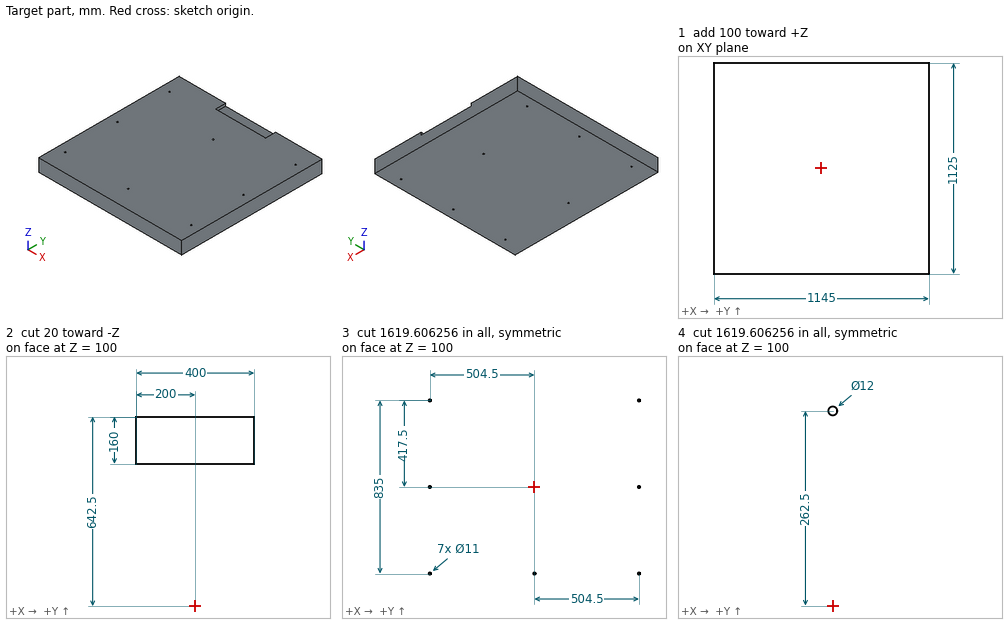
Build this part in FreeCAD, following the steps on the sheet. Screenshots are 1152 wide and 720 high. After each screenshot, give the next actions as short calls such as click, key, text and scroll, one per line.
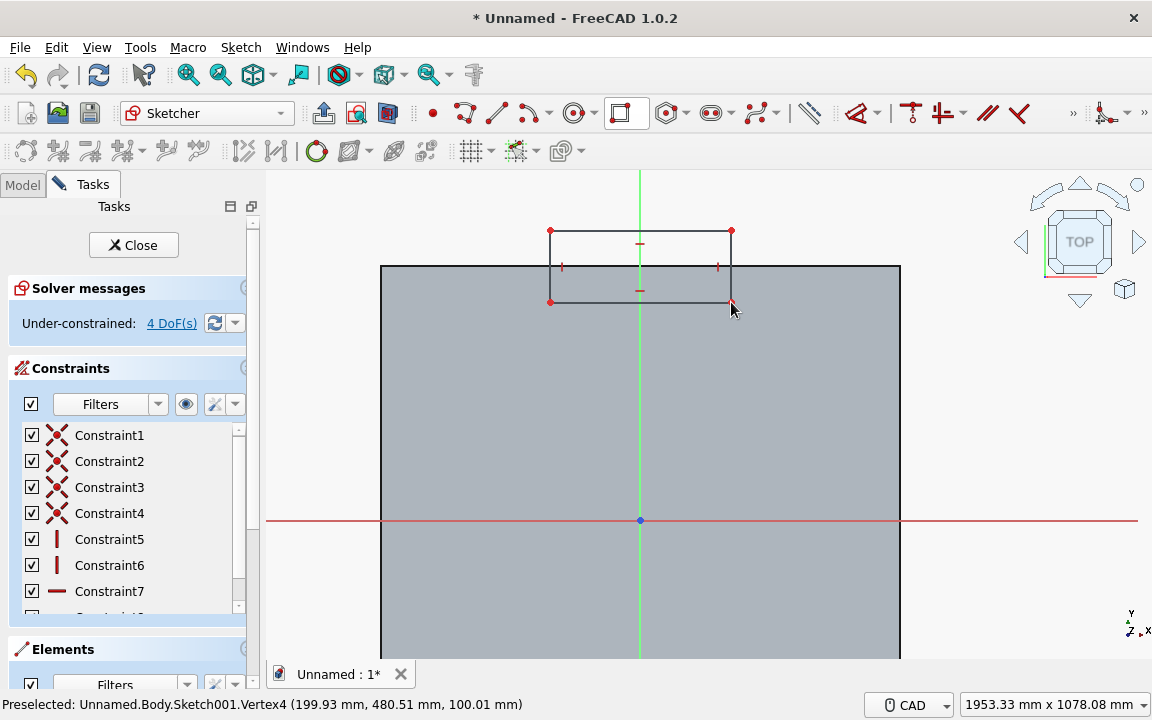
key(d)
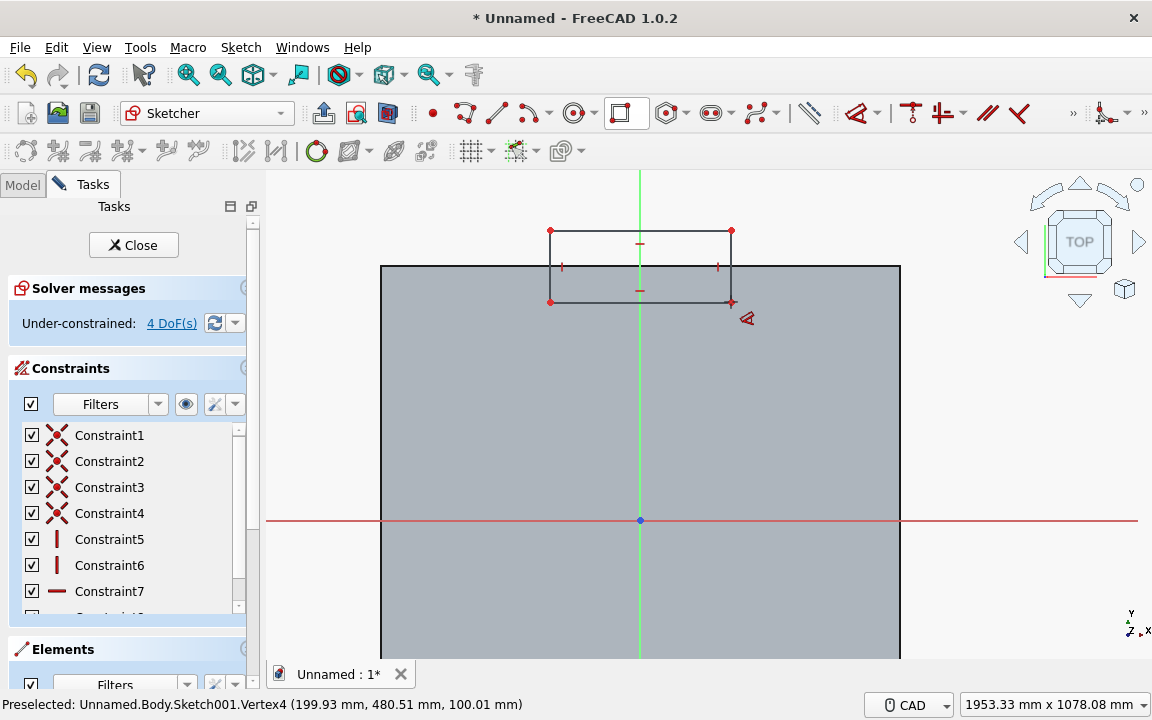
click(550, 253)
click(516, 267)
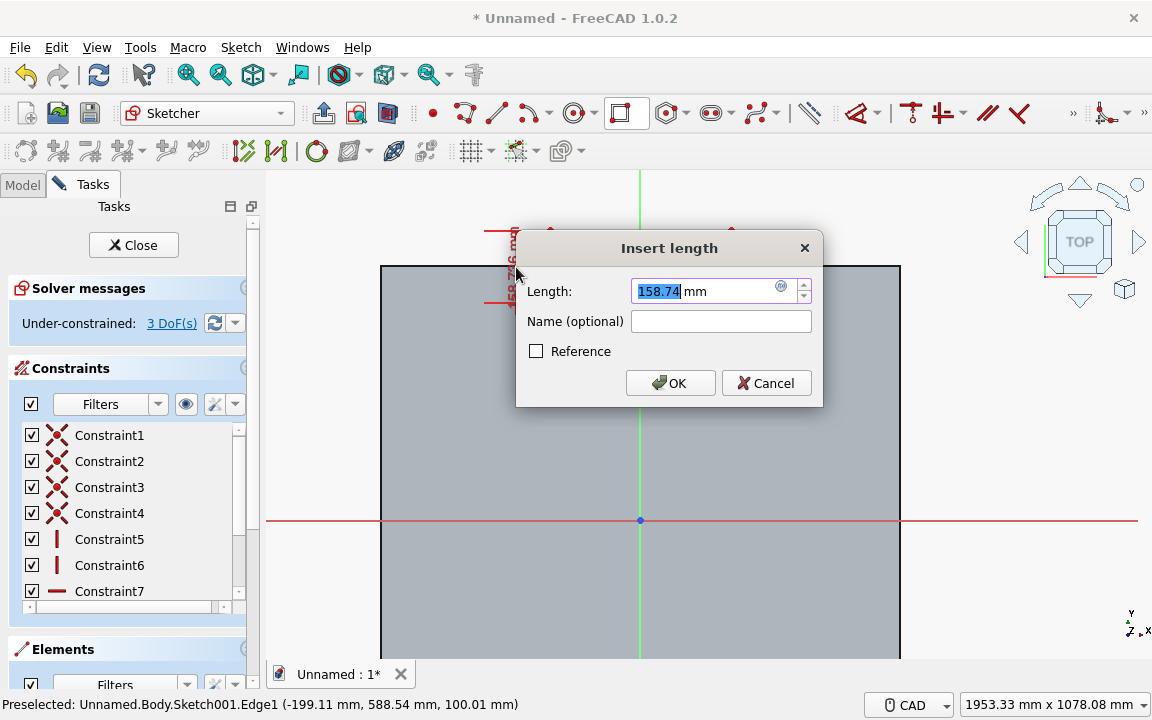
text(160)
key(Return)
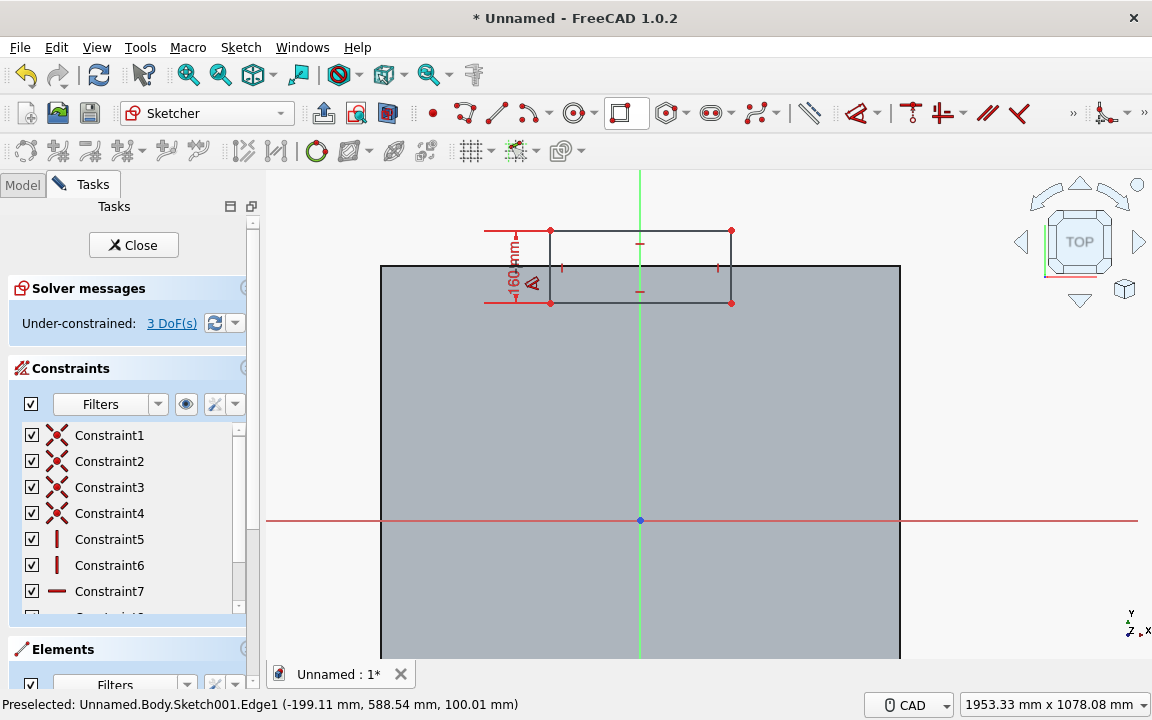
click(604, 303)
click(599, 269)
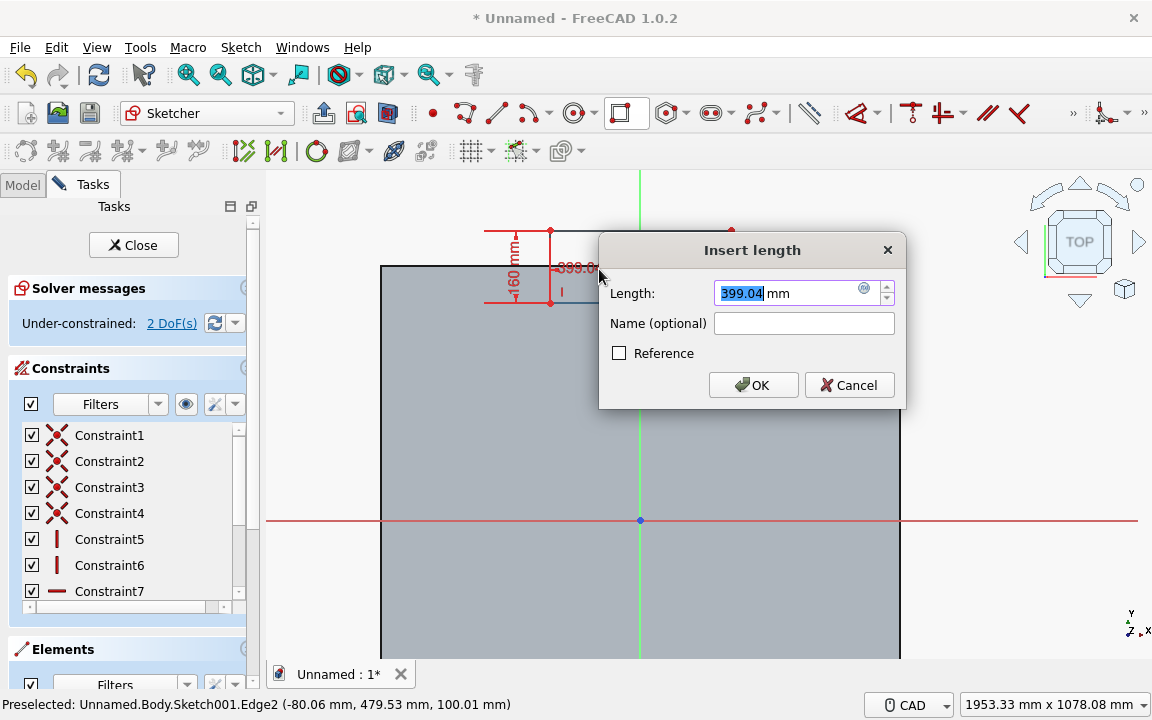
text(400)
key(Return)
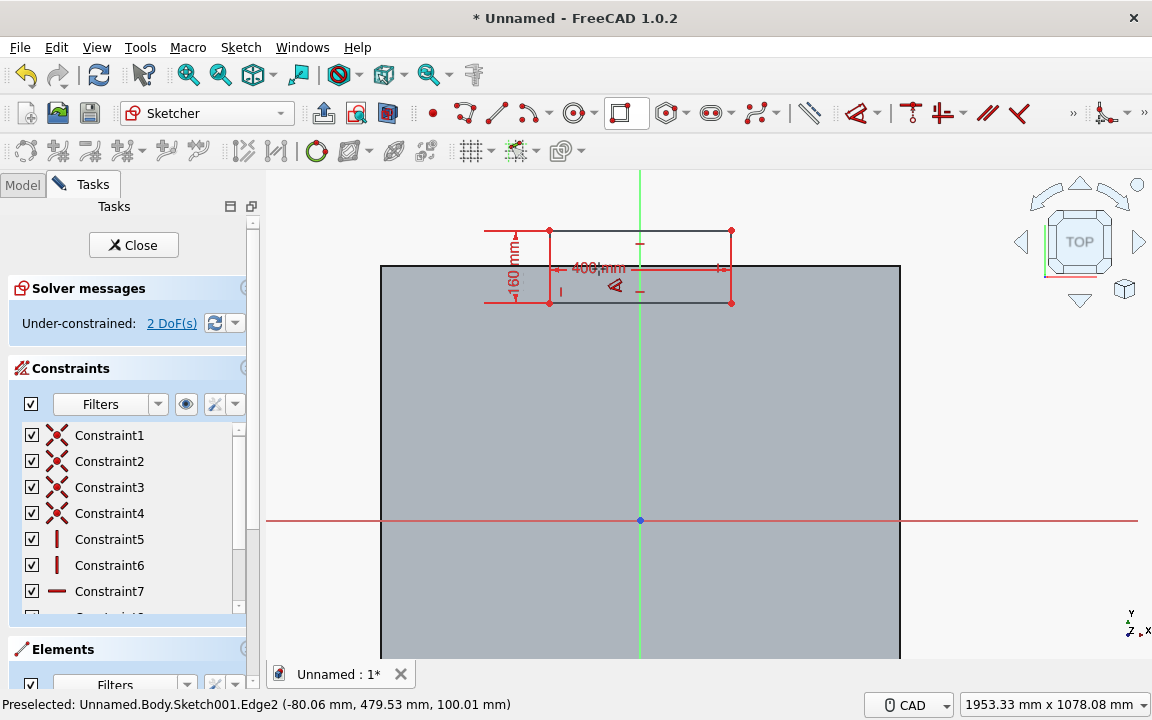
click(550, 231)
click(595, 555)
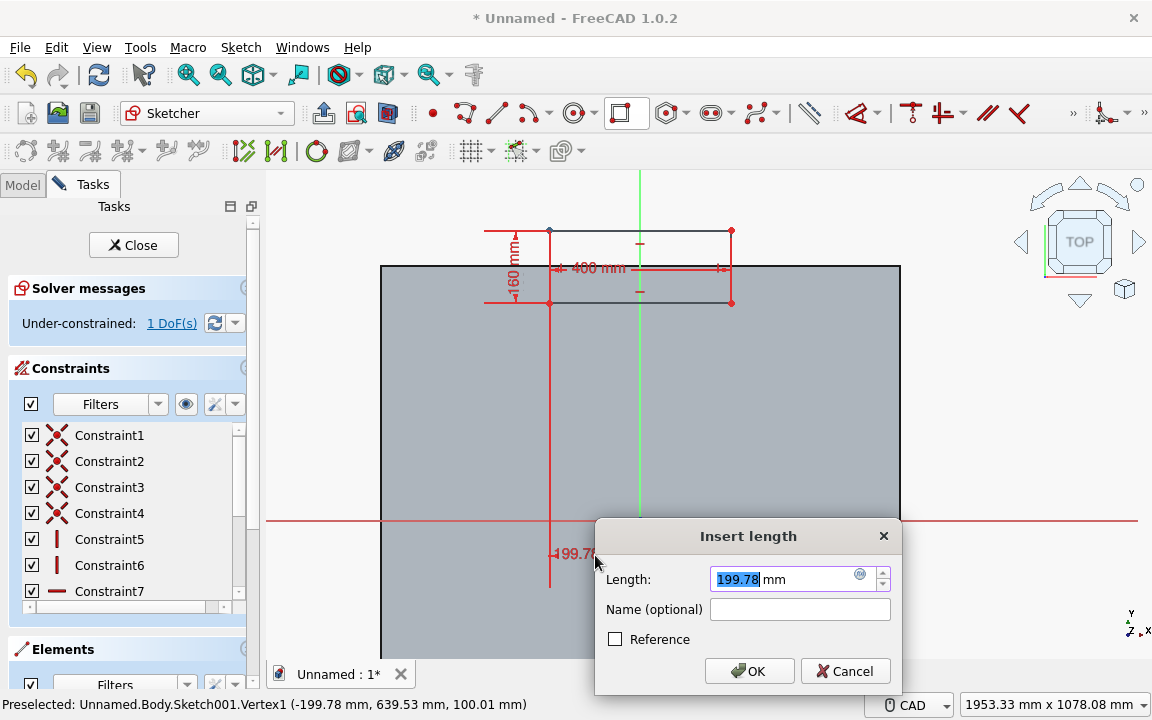
text(200)
key(Return)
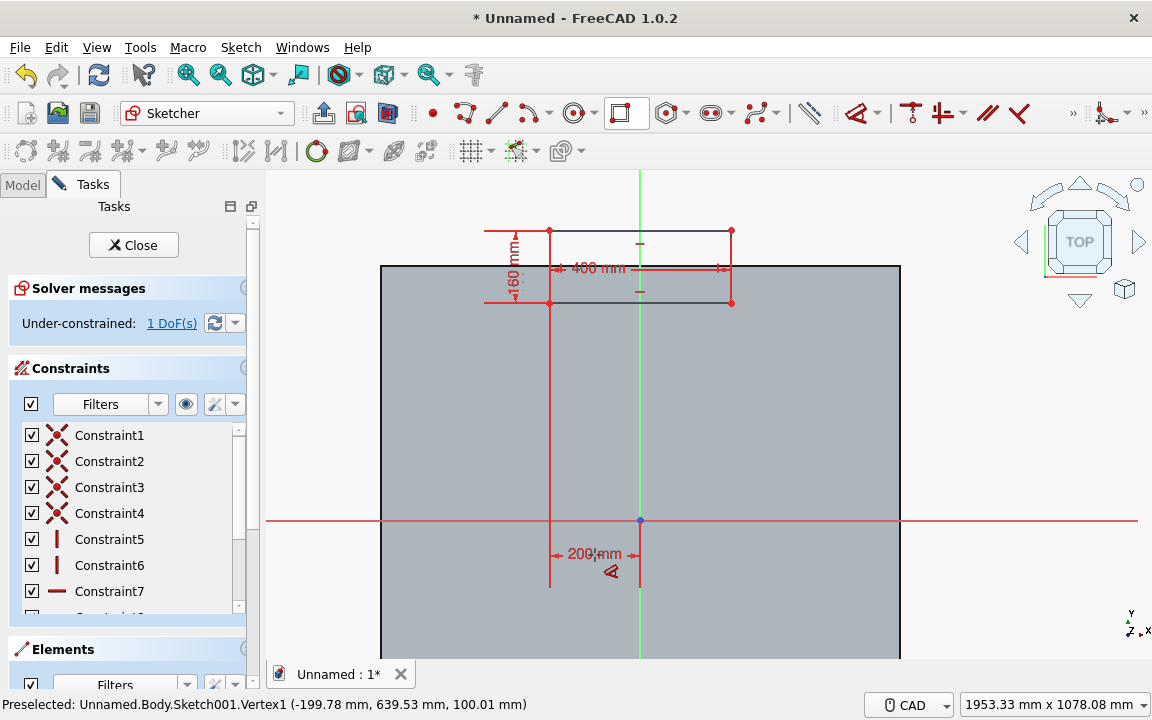
click(550, 231)
click(516, 376)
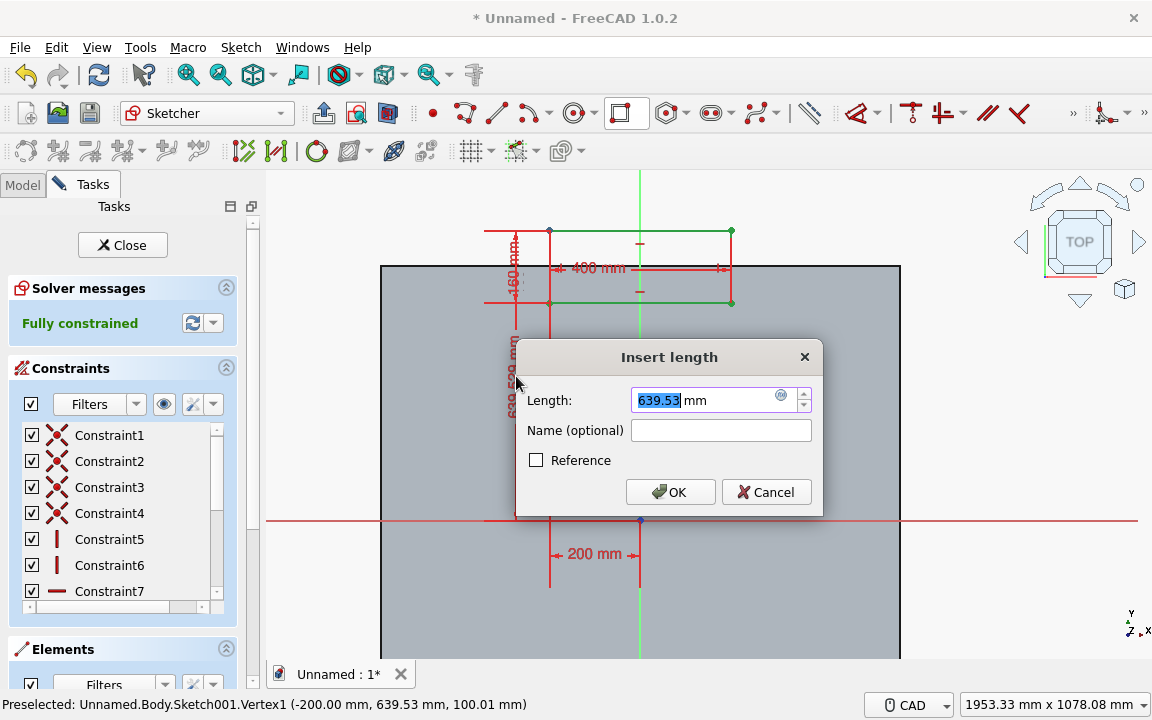
text(642.5)
key(Return)
key(Escape)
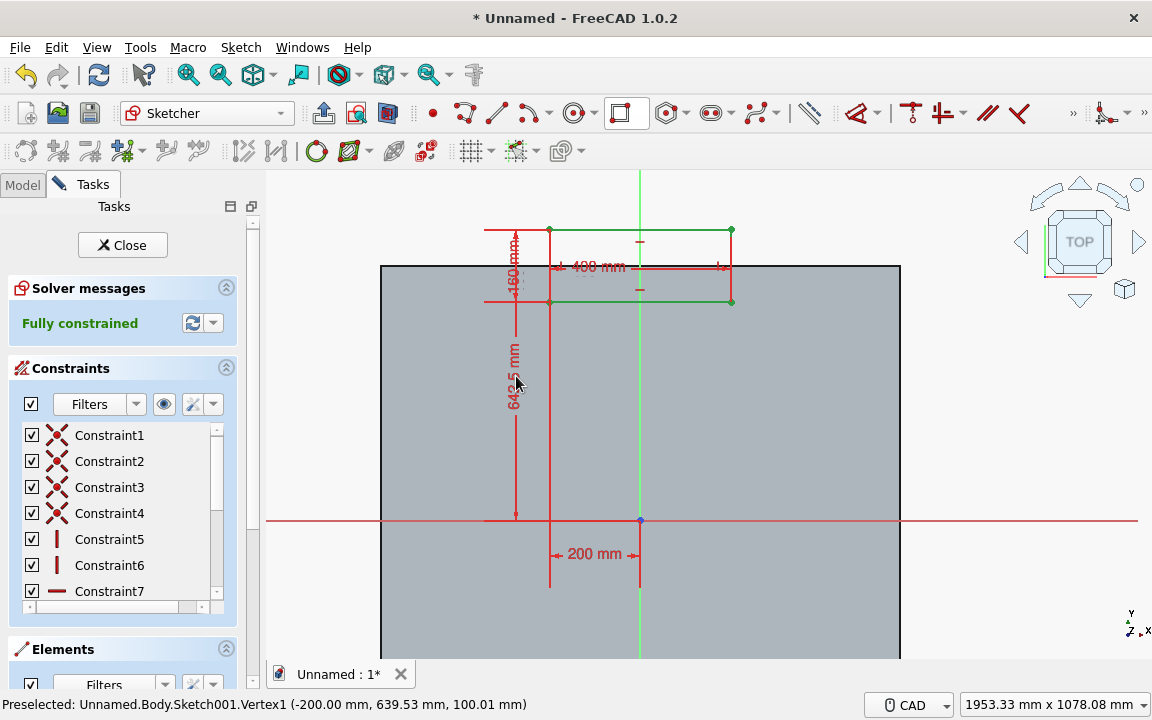
click(123, 245)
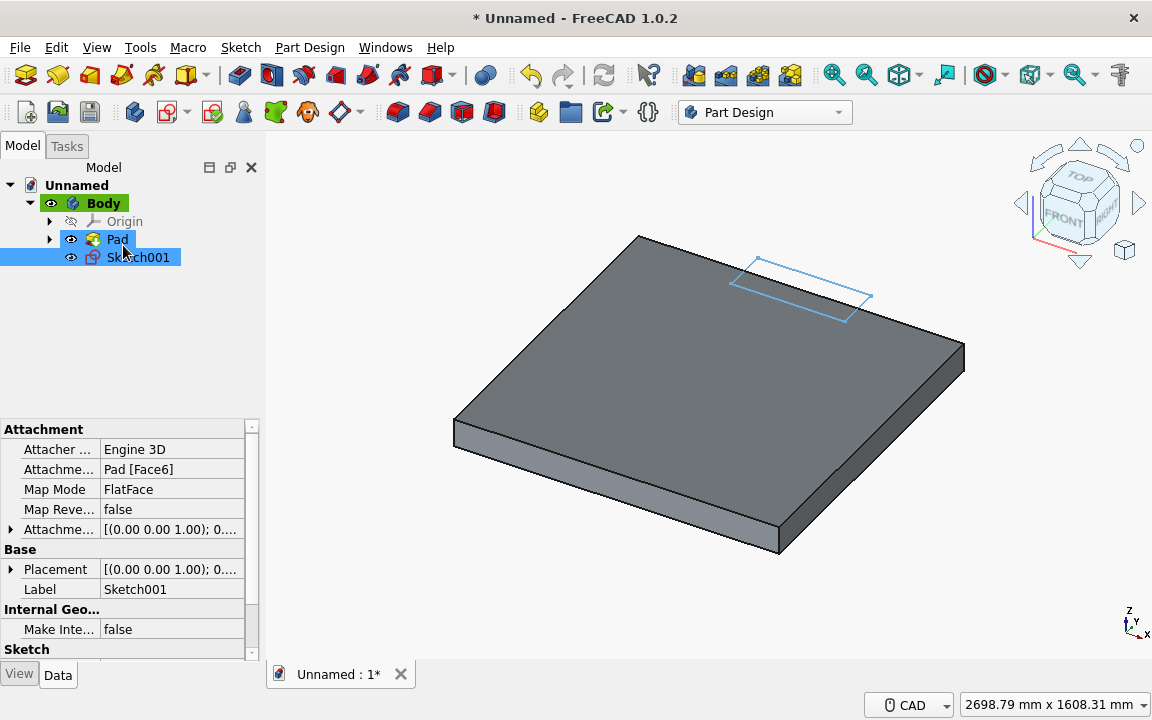
click(240, 76)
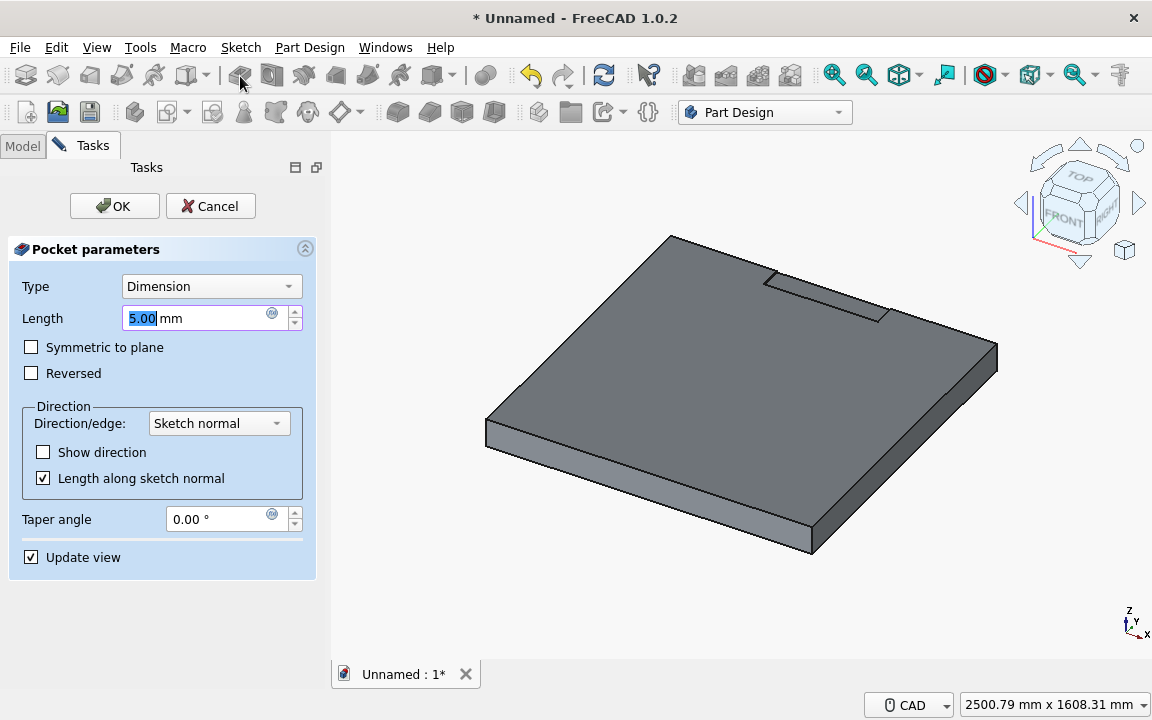
text(20)
key(Tab)